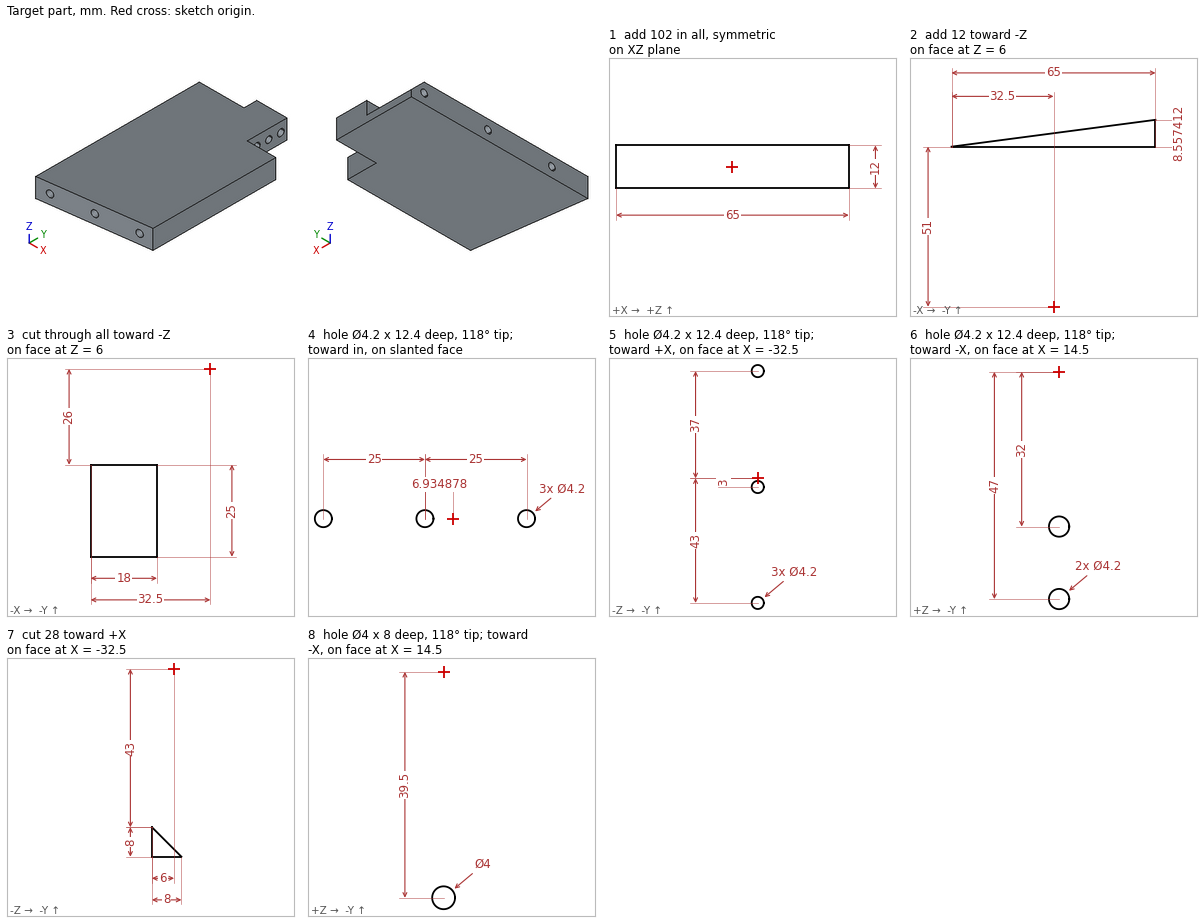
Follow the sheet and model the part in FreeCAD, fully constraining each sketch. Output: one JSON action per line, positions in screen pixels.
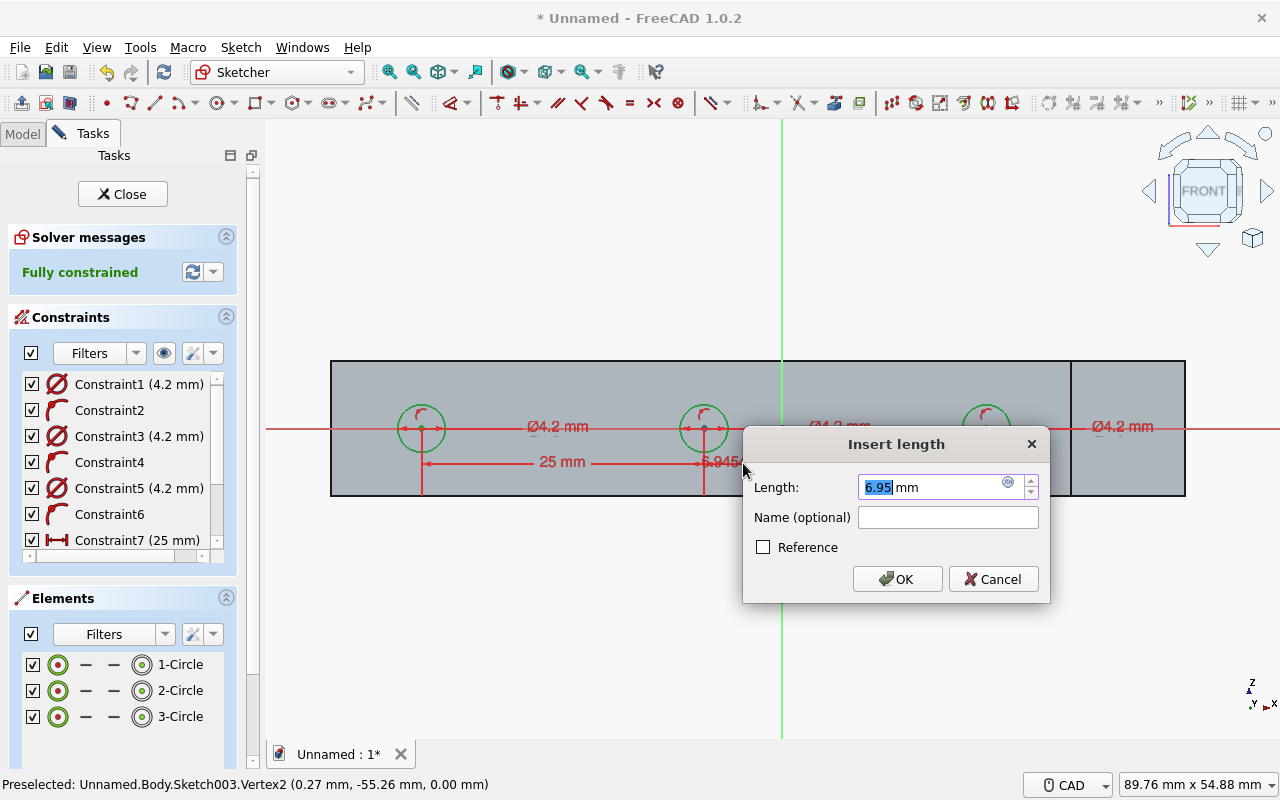
{"action": "type", "text": "6.934878"}
{"action": "key", "text": "Return"}
{"action": "key", "text": "Escape"}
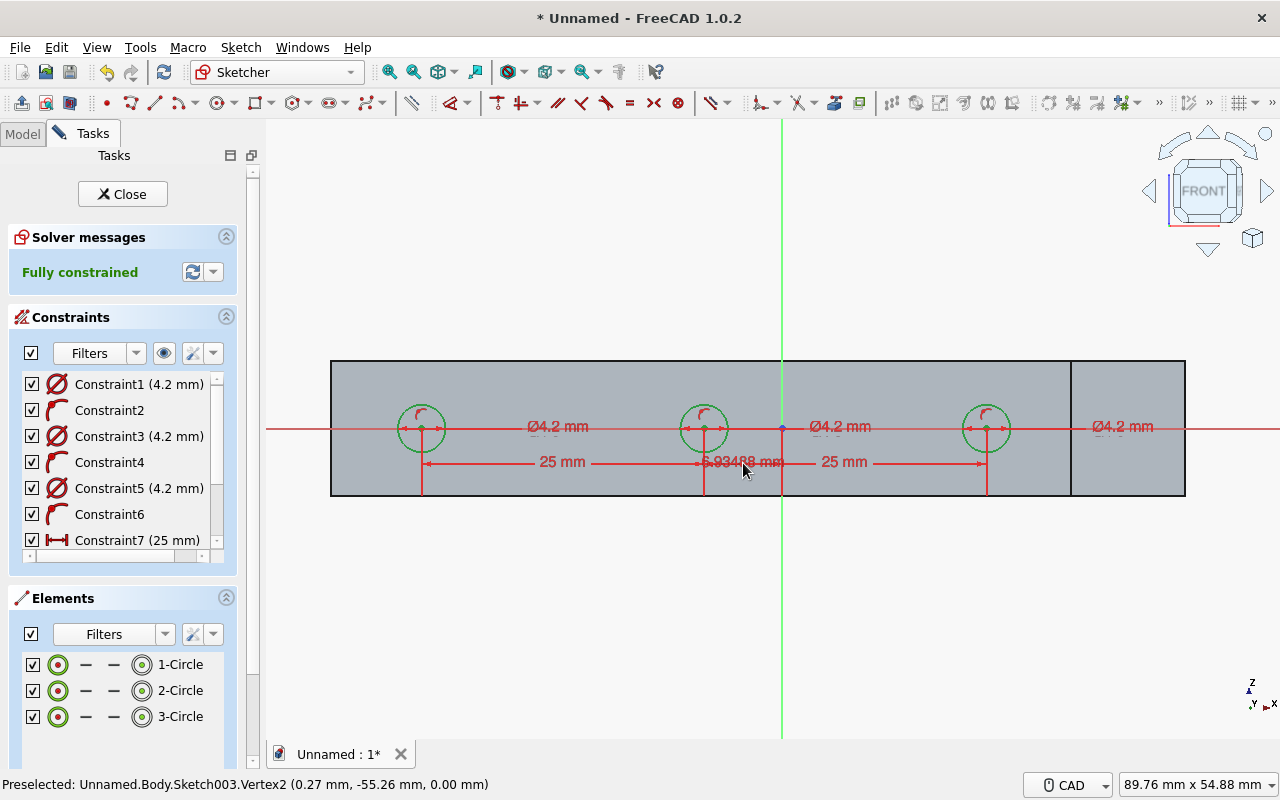
{"action": "left_click", "coordinate": [123, 194]}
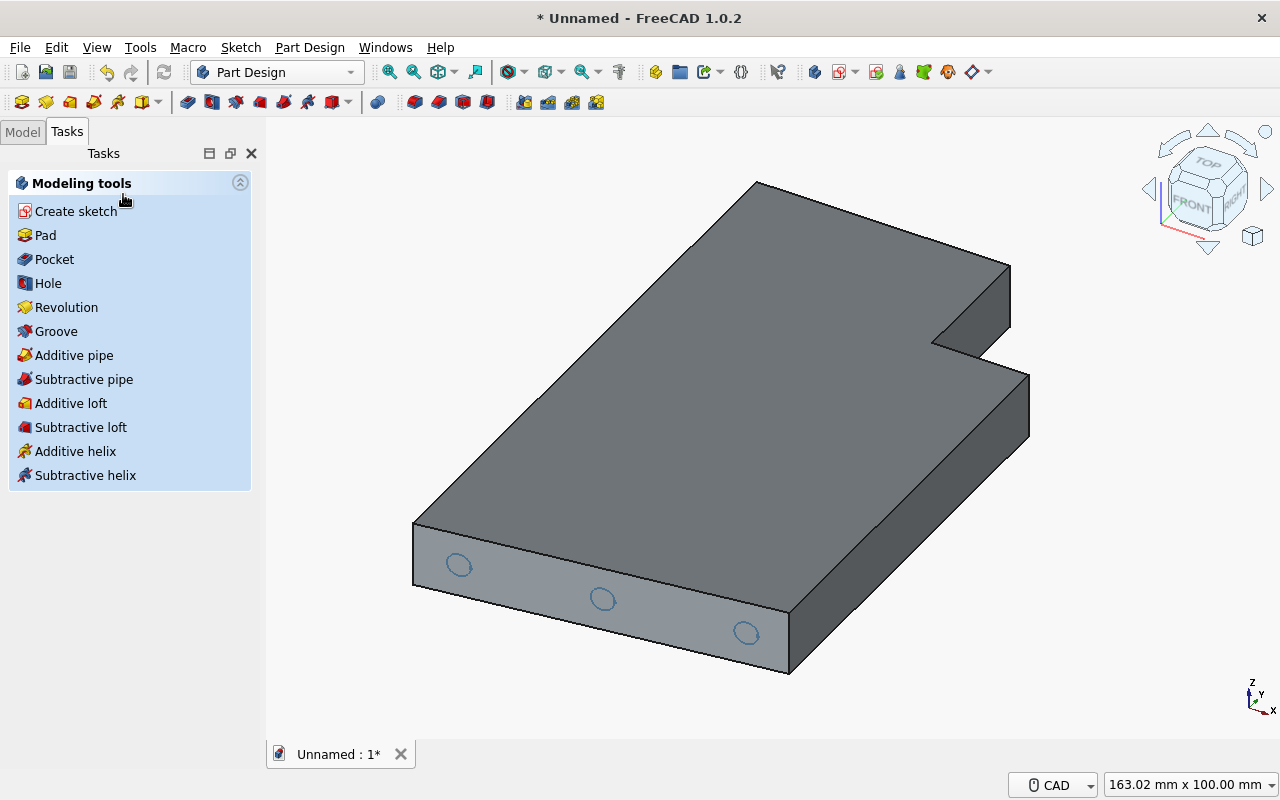
{"action": "left_click", "coordinate": [212, 102]}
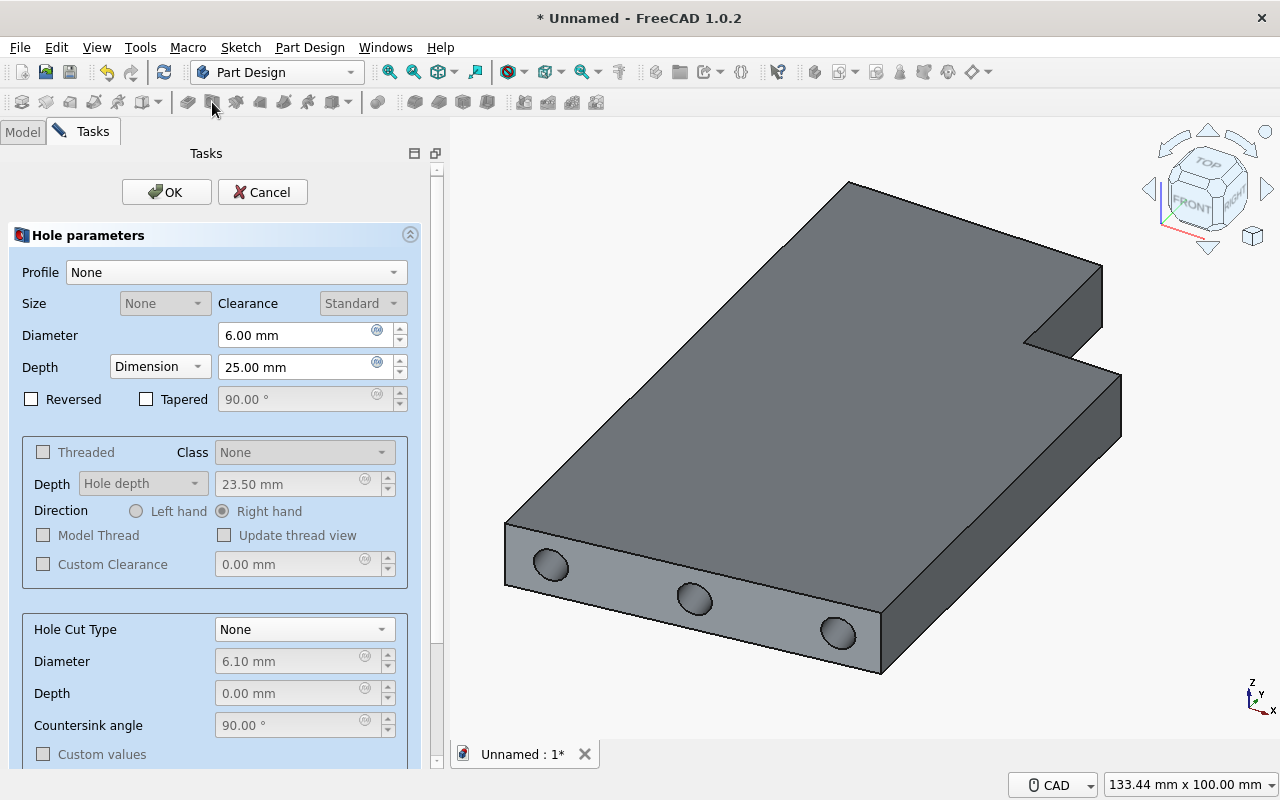
{"action": "triple_click", "coordinate": [305, 335]}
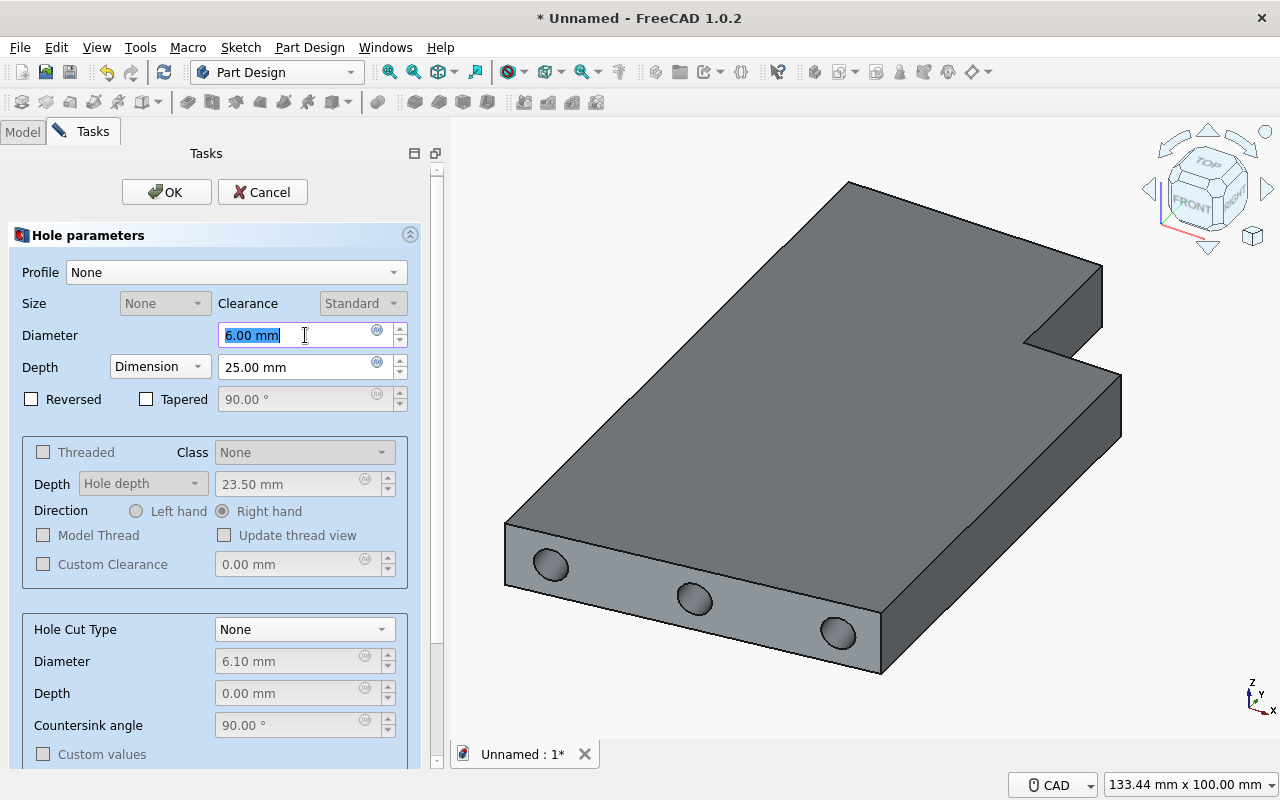
{"action": "type", "text": "4.2"}
{"action": "key", "text": "Tab"}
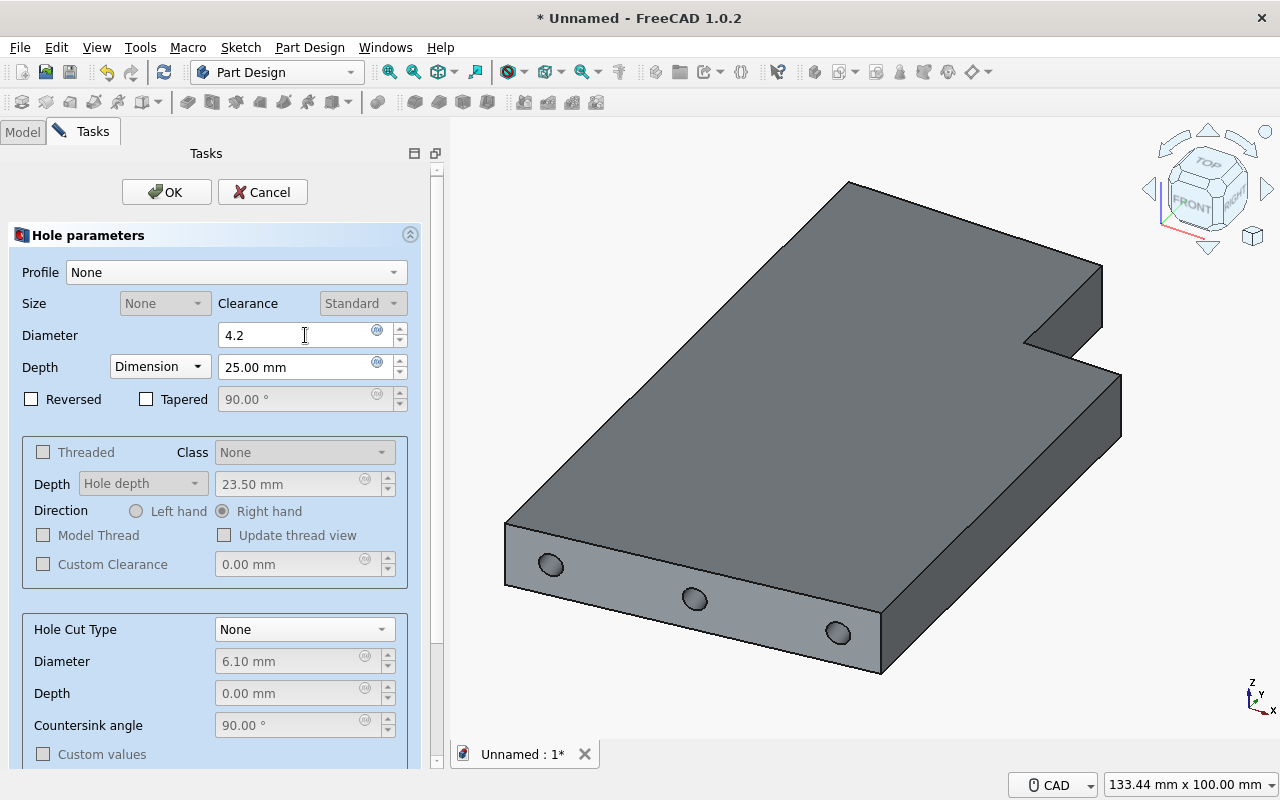
{"action": "triple_click", "coordinate": [305, 367]}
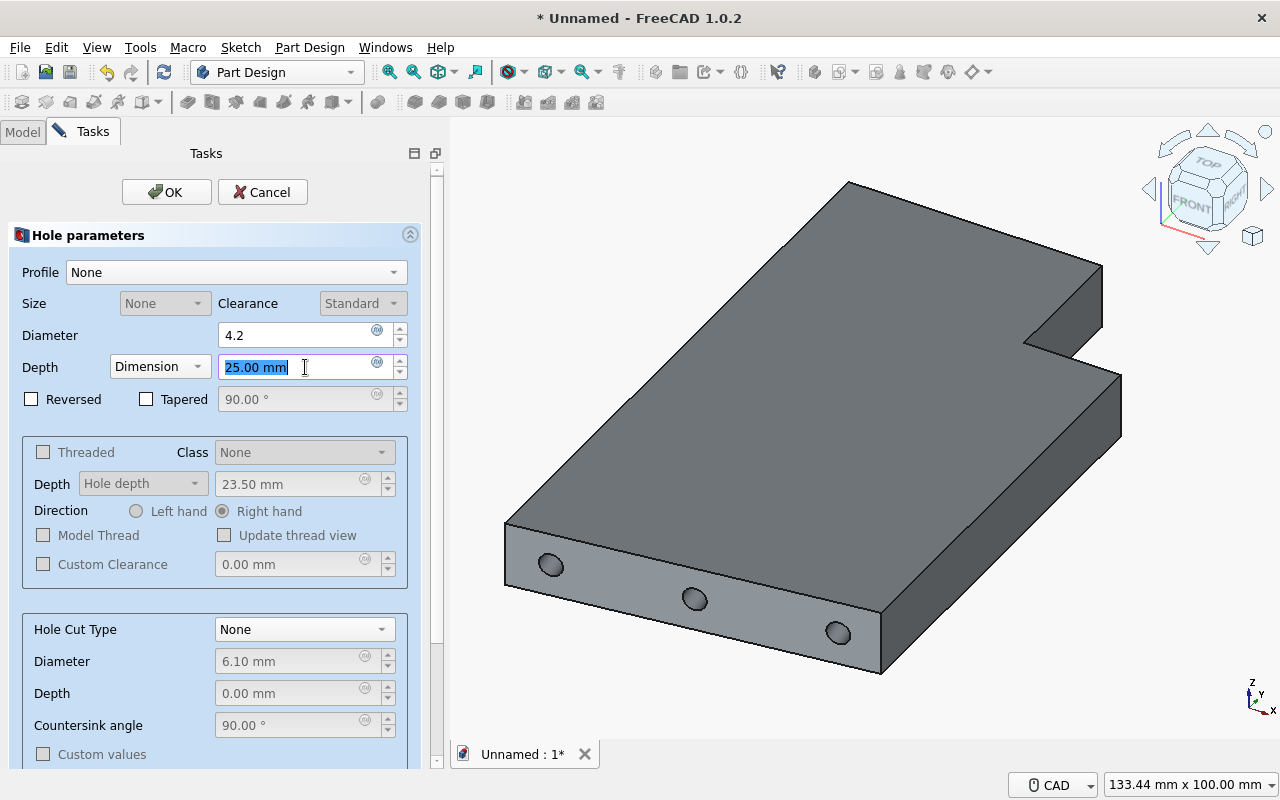
{"action": "type", "text": "12.4"}
{"action": "key", "text": "Tab"}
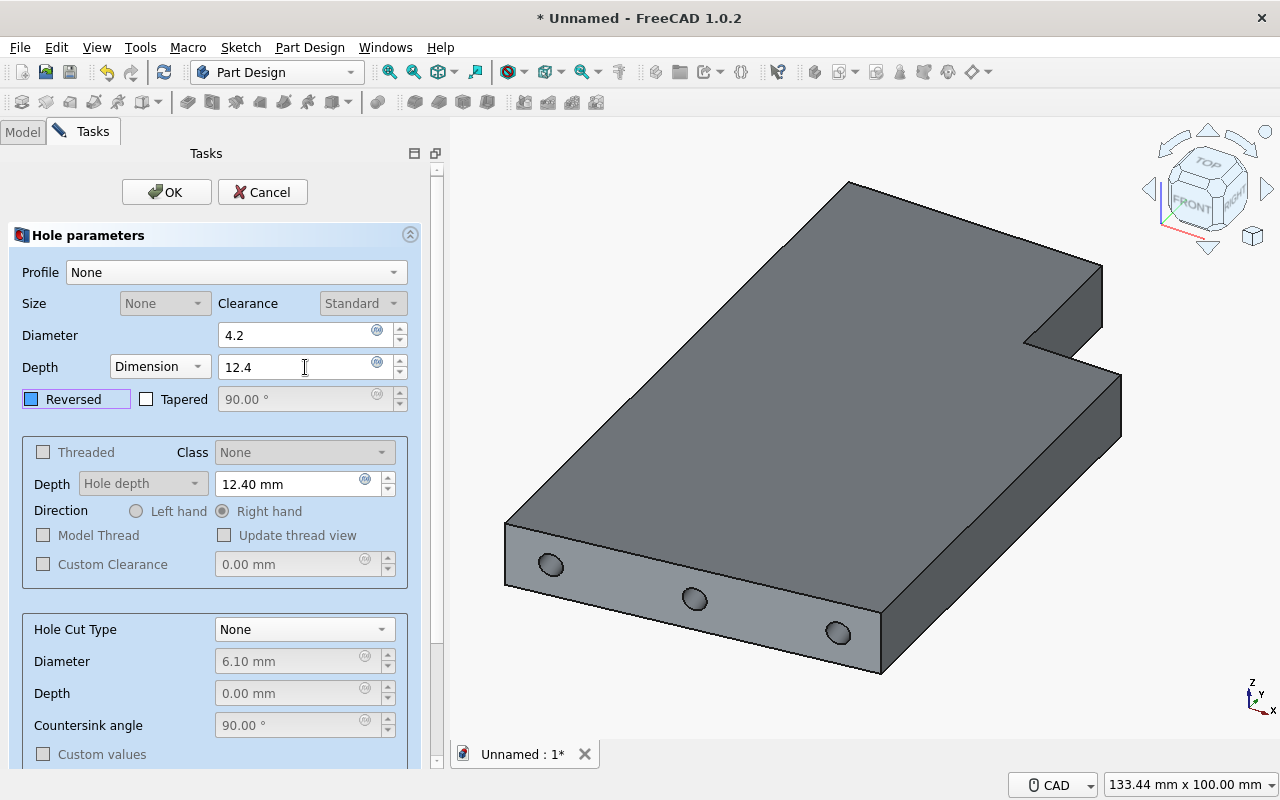
{"action": "left_click", "coordinate": [167, 192]}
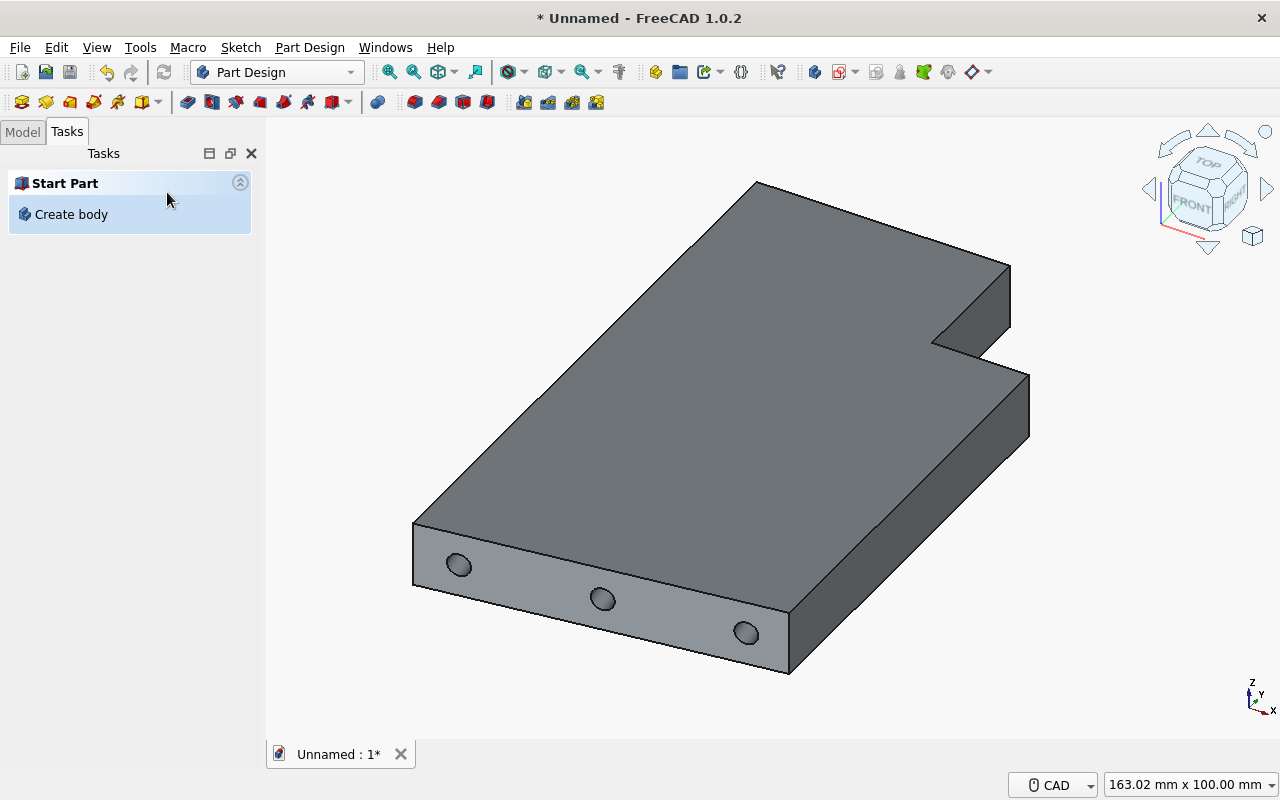
{"action": "key", "text": "6"}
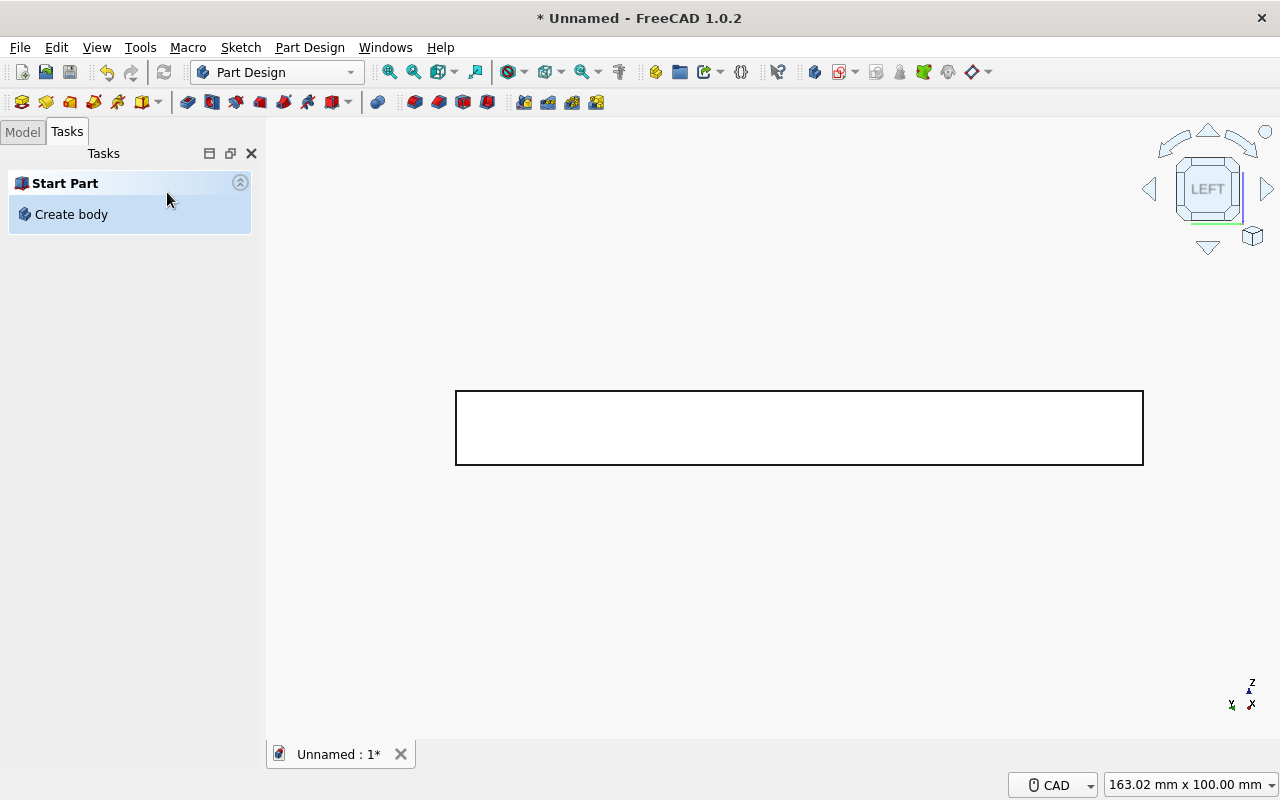
{"action": "left_click", "coordinate": [603, 427]}